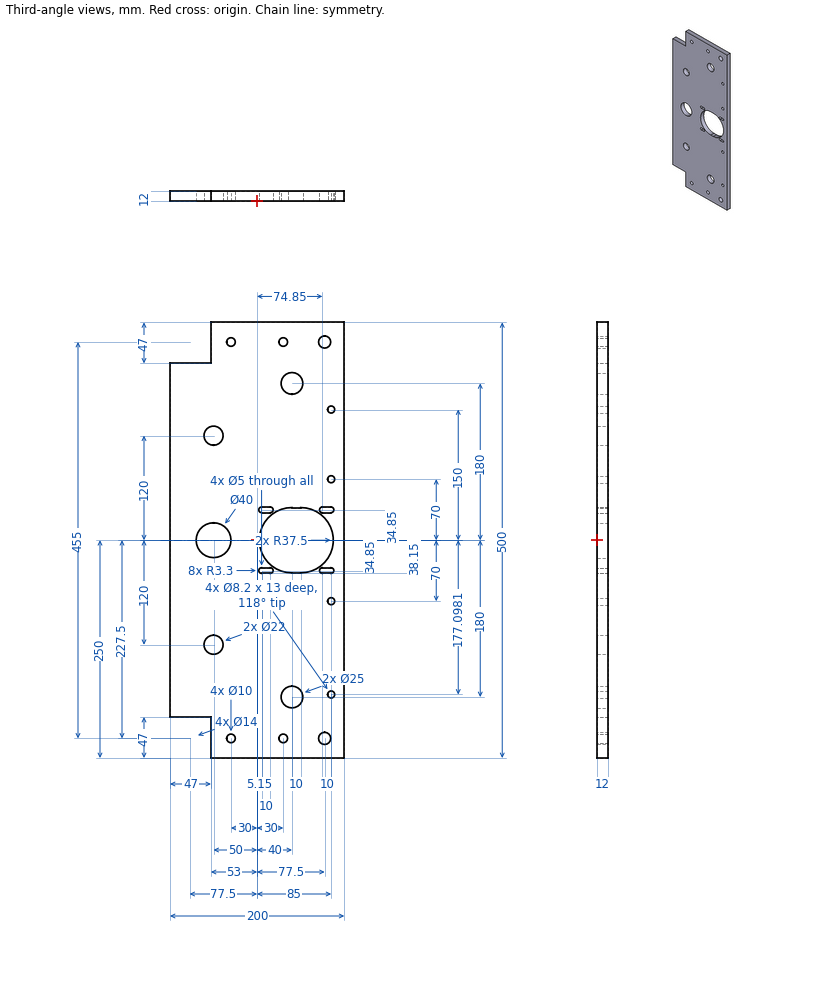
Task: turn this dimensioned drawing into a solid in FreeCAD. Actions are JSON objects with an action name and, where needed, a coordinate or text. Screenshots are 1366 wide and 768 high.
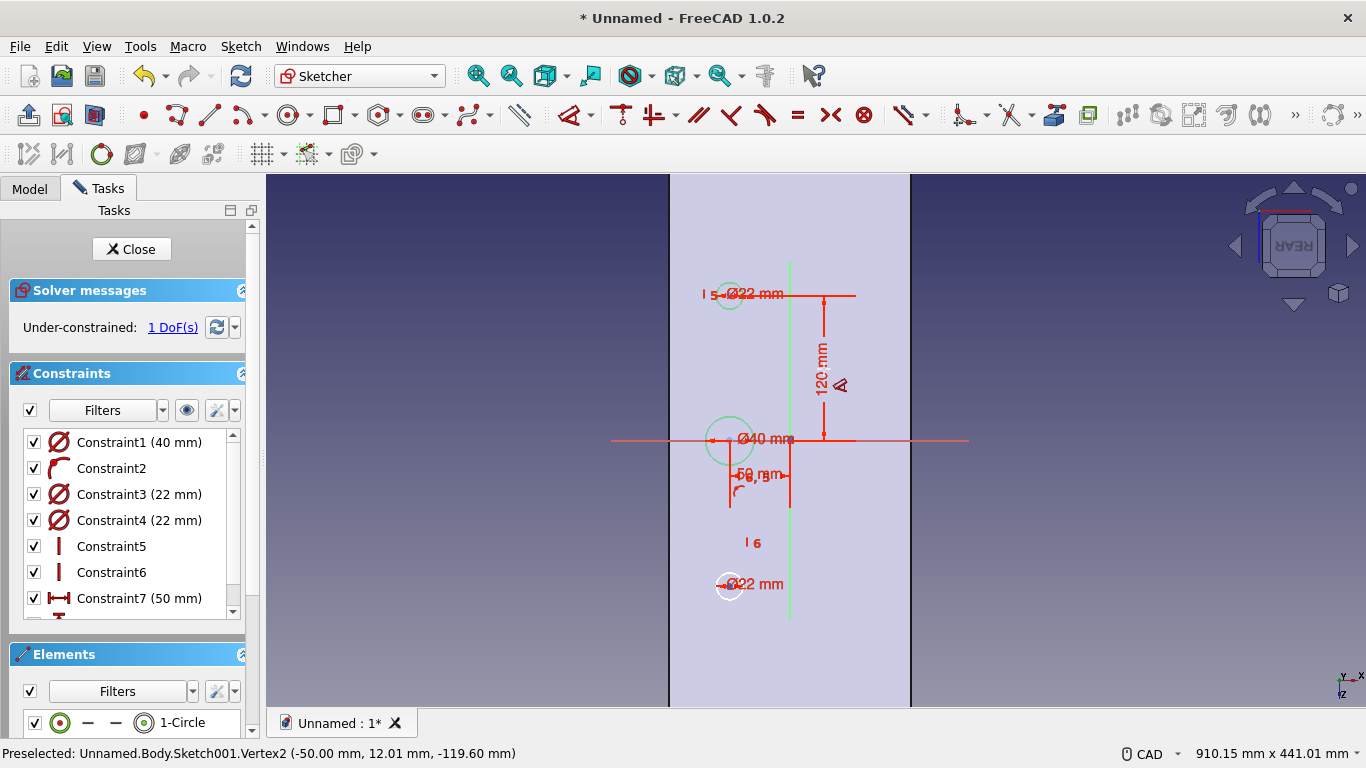
{"action": "left_click", "coordinate": [730, 586]}
{"action": "left_click", "coordinate": [824, 514]}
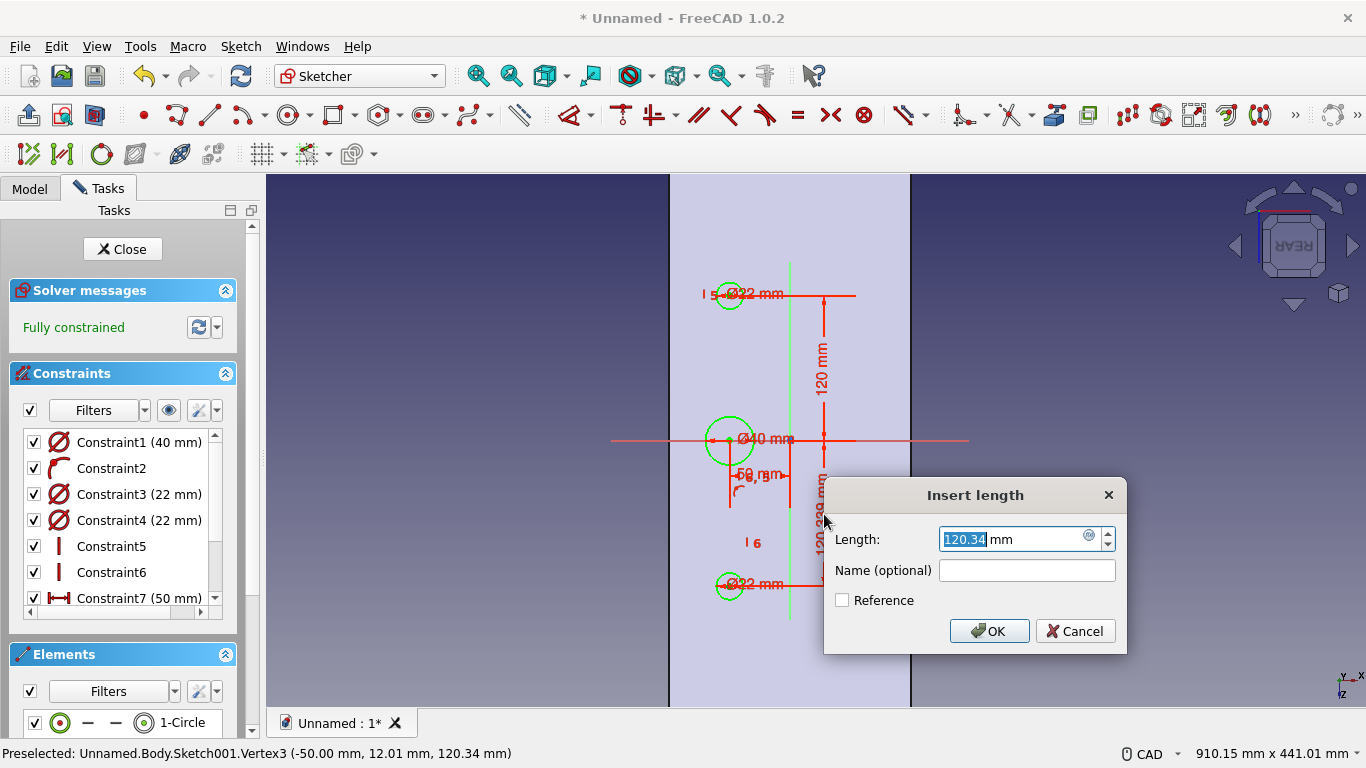
{"action": "type", "text": "120"}
{"action": "key", "text": "Return"}
{"action": "key", "text": "Escape"}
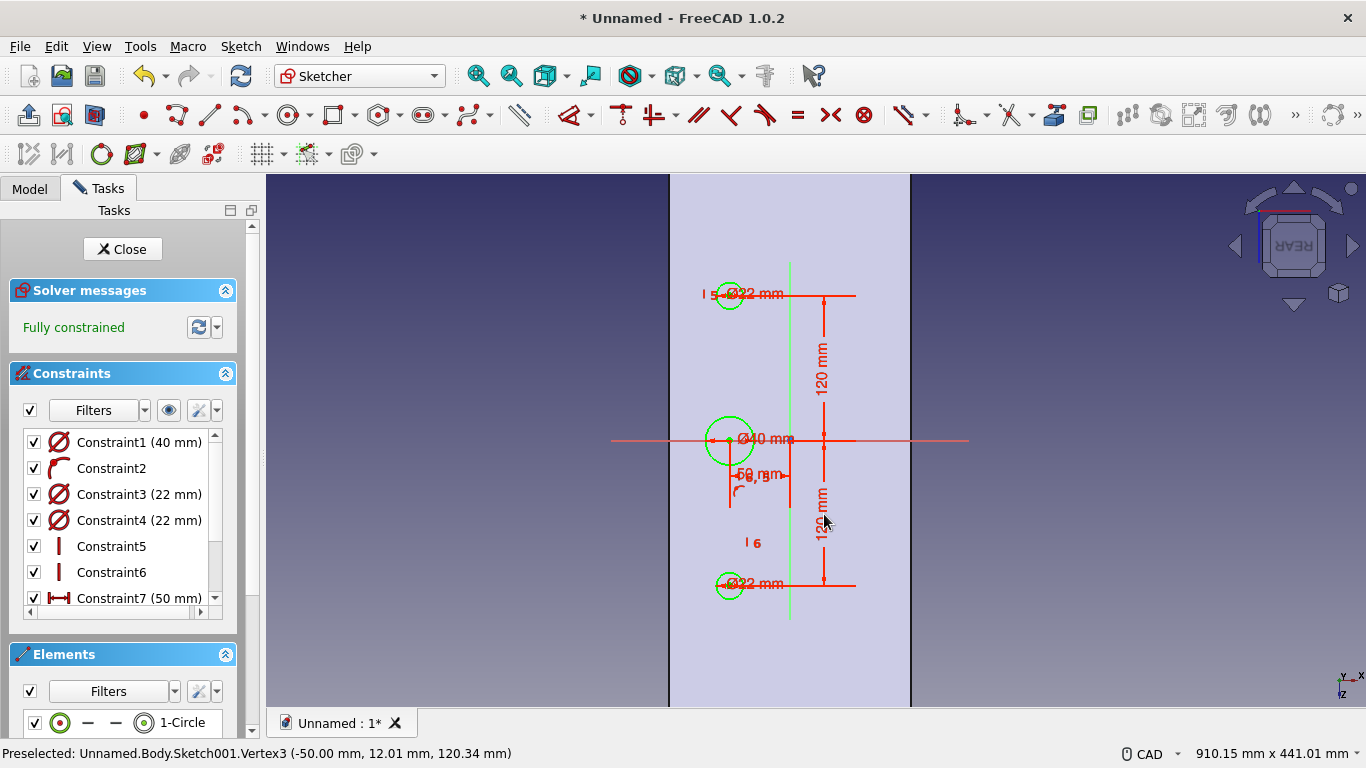
{"action": "left_click", "coordinate": [123, 249]}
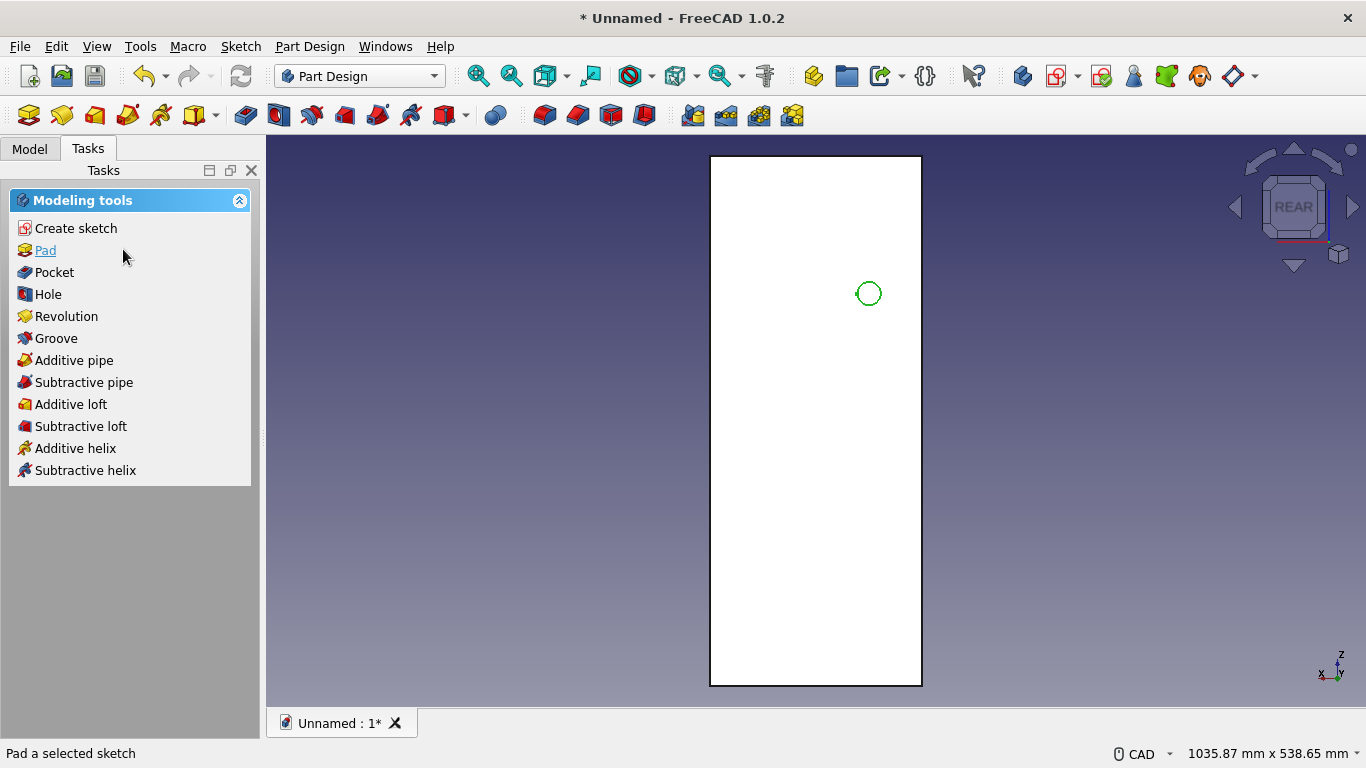
{"action": "left_click", "coordinate": [246, 116]}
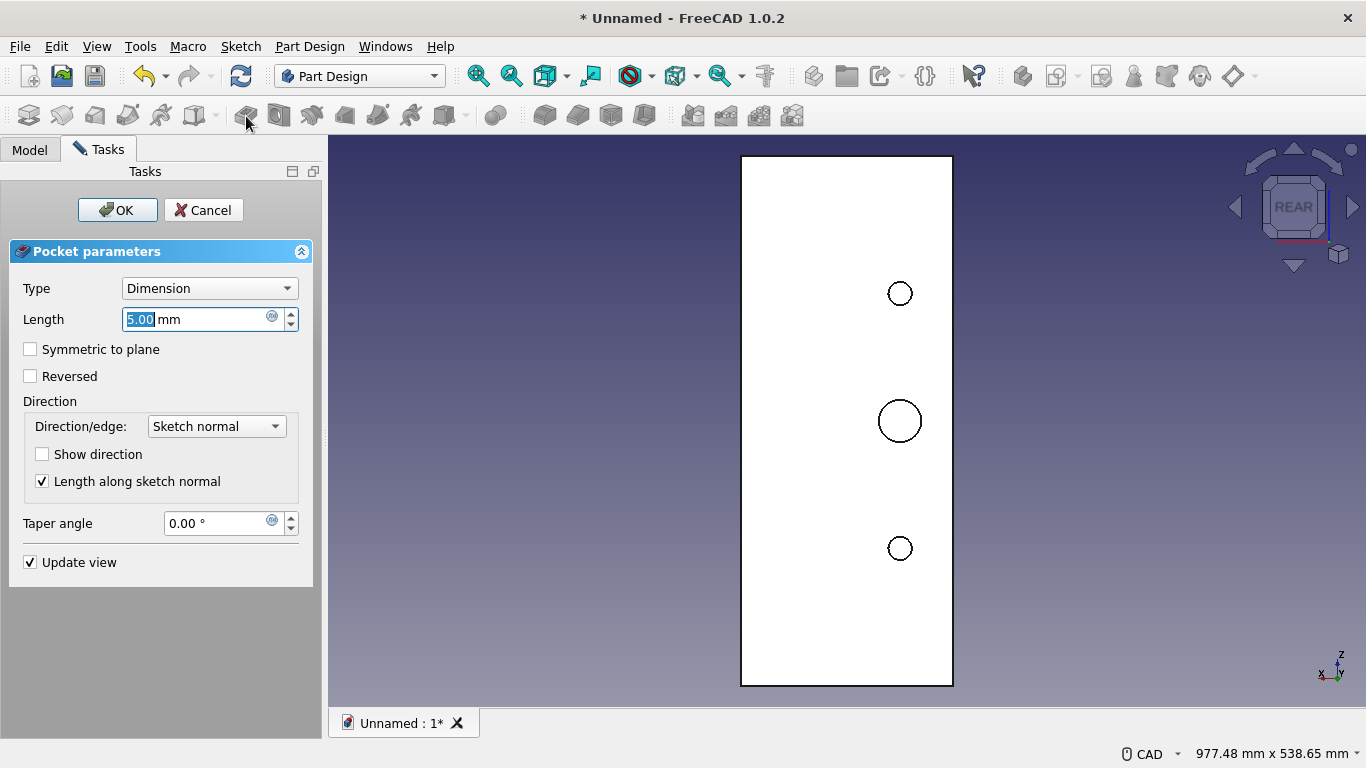
{"action": "type", "text": "12"}
{"action": "key", "text": "Tab"}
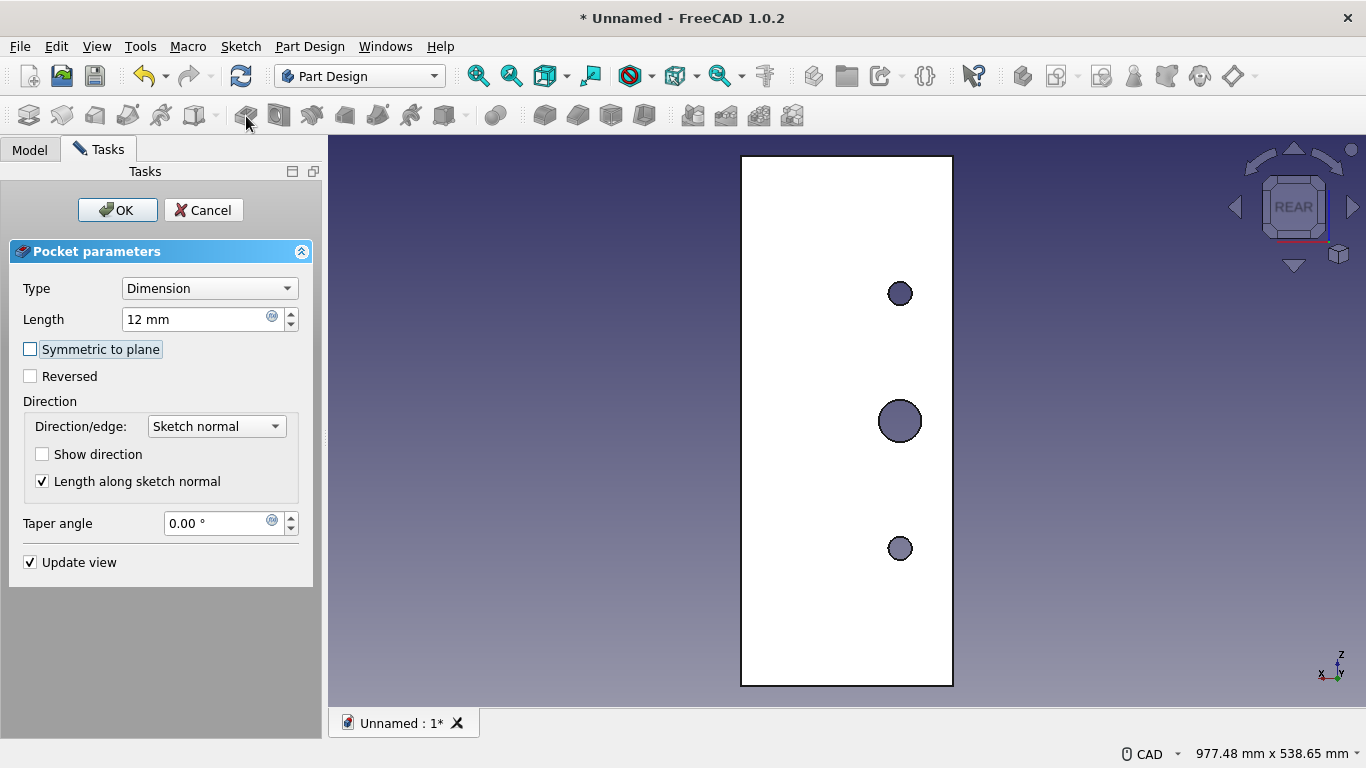
{"action": "left_click", "coordinate": [118, 210]}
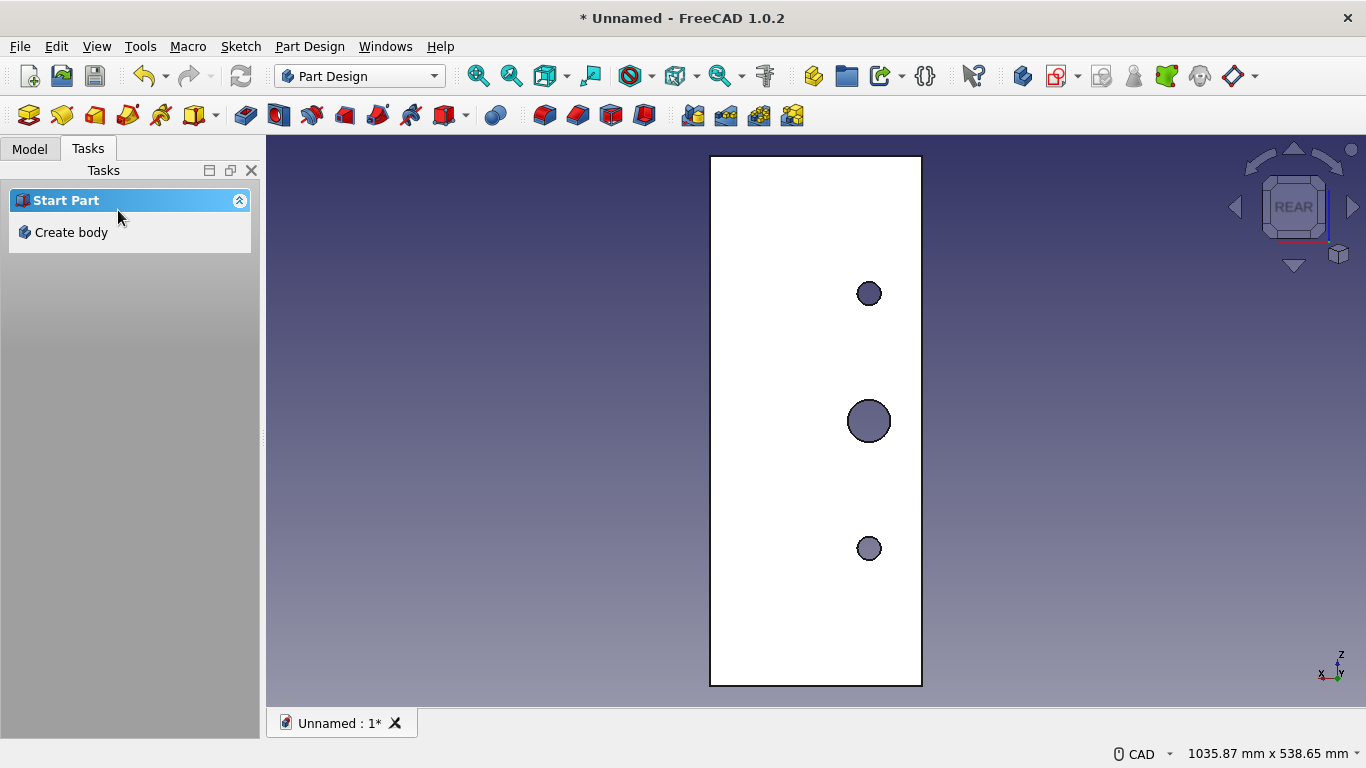
{"action": "left_click", "coordinate": [786, 344]}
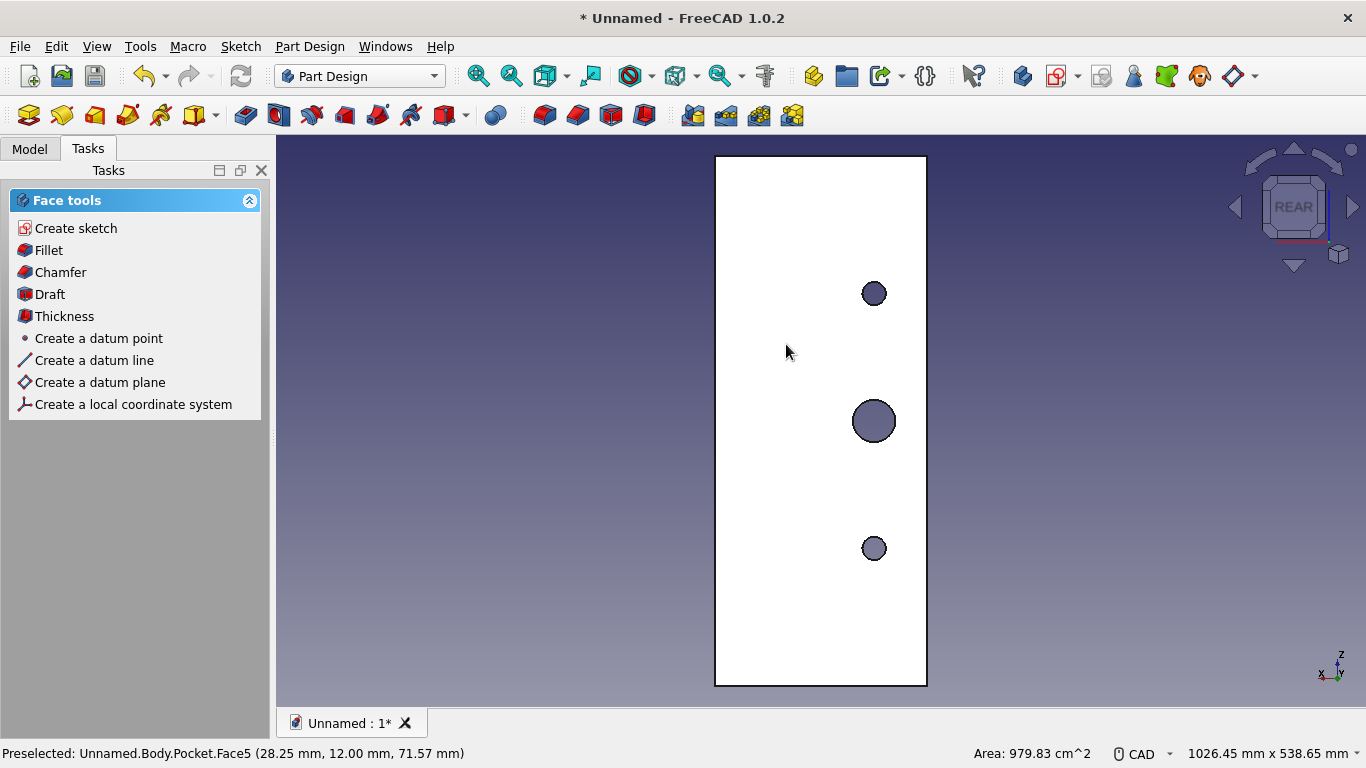
{"action": "left_click", "coordinate": [1056, 76]}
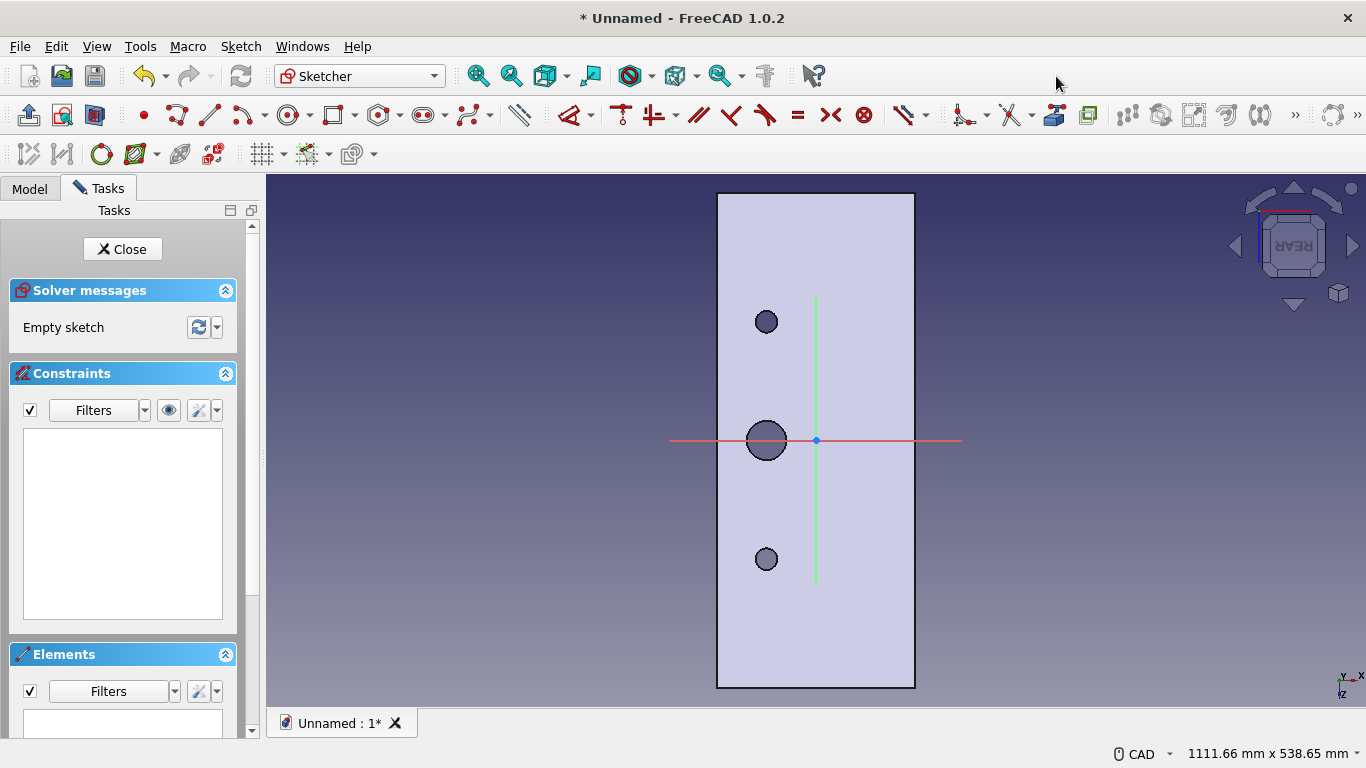
{"action": "key", "text": "g c"}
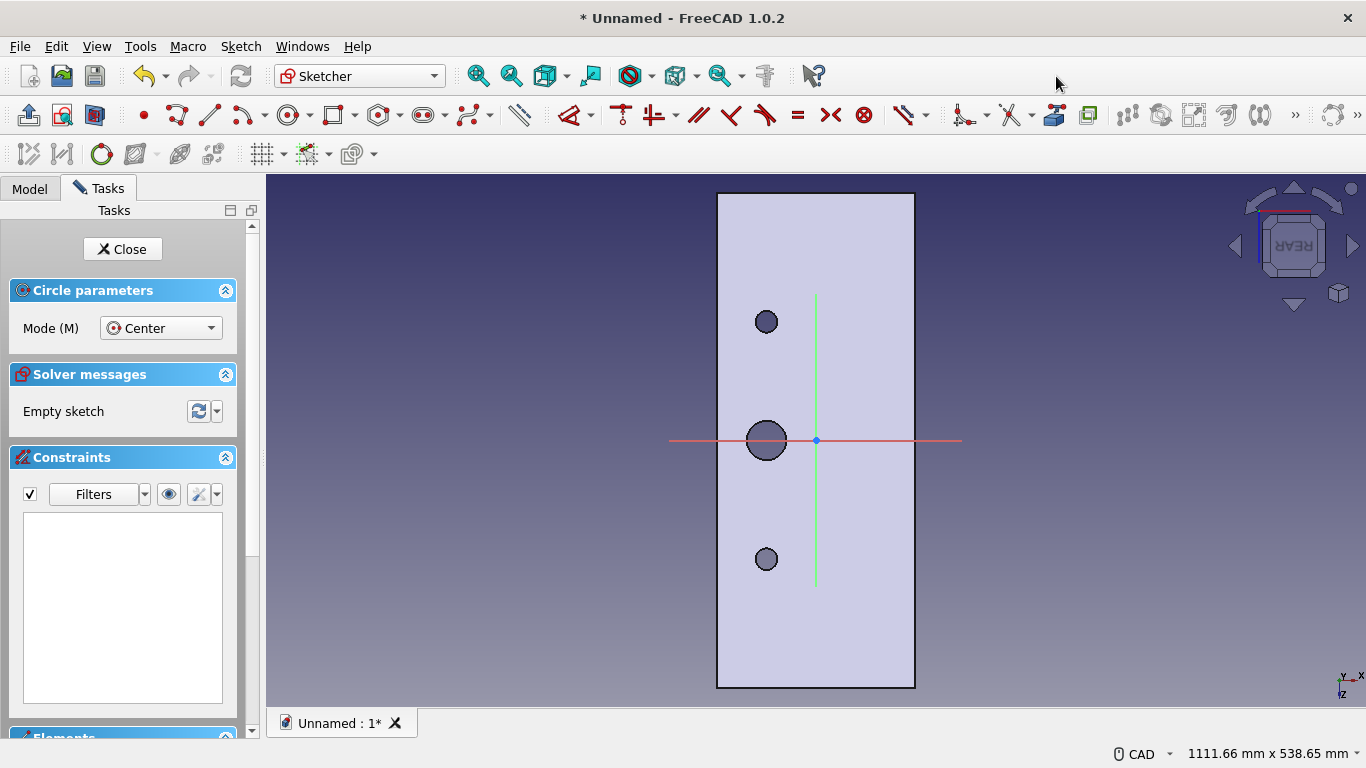
{"action": "scroll", "coordinate": [856, 262], "scroll_direction": "up", "scroll_amount": 4}